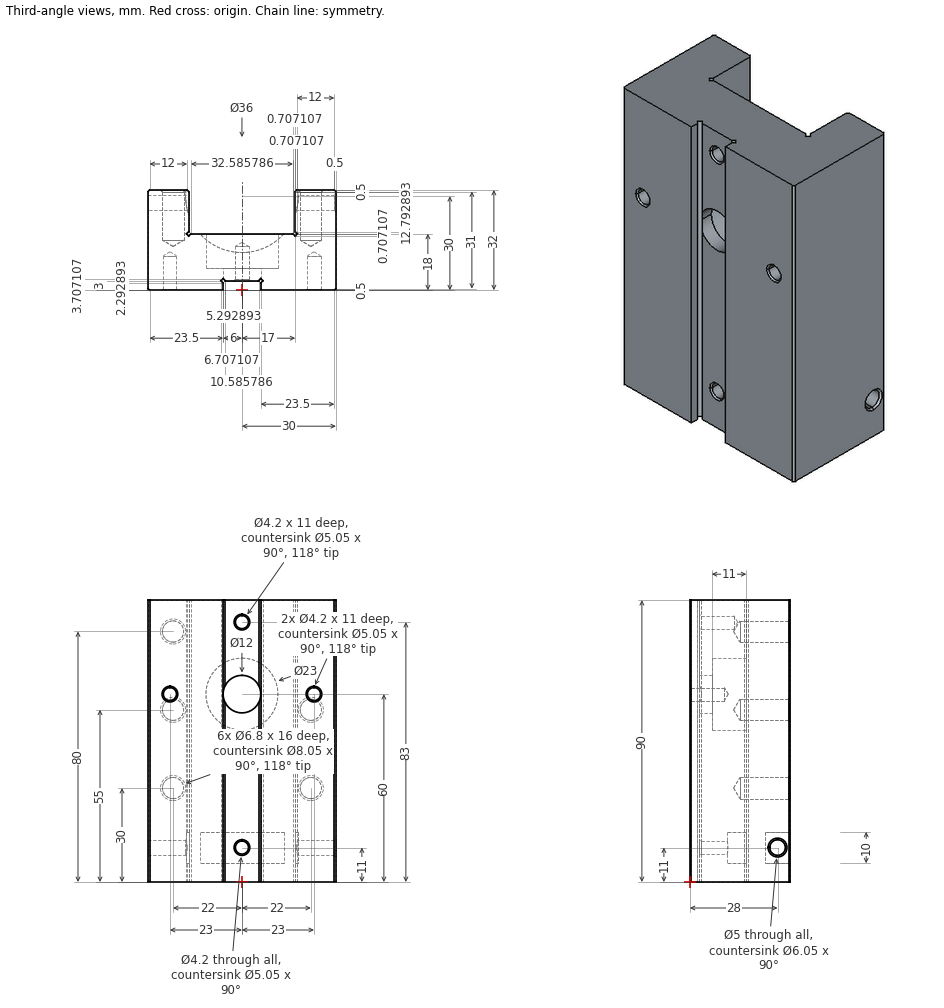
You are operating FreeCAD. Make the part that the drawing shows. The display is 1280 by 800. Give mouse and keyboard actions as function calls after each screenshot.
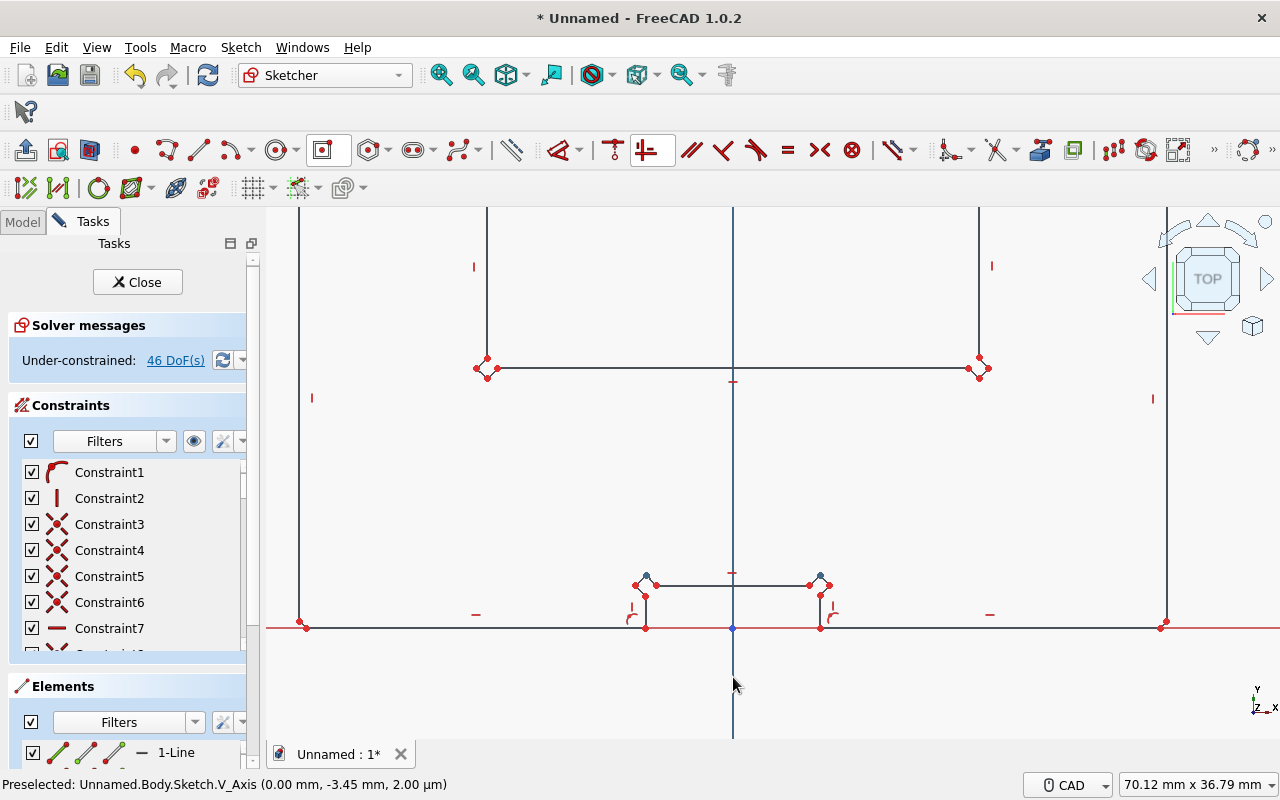
click(820, 150)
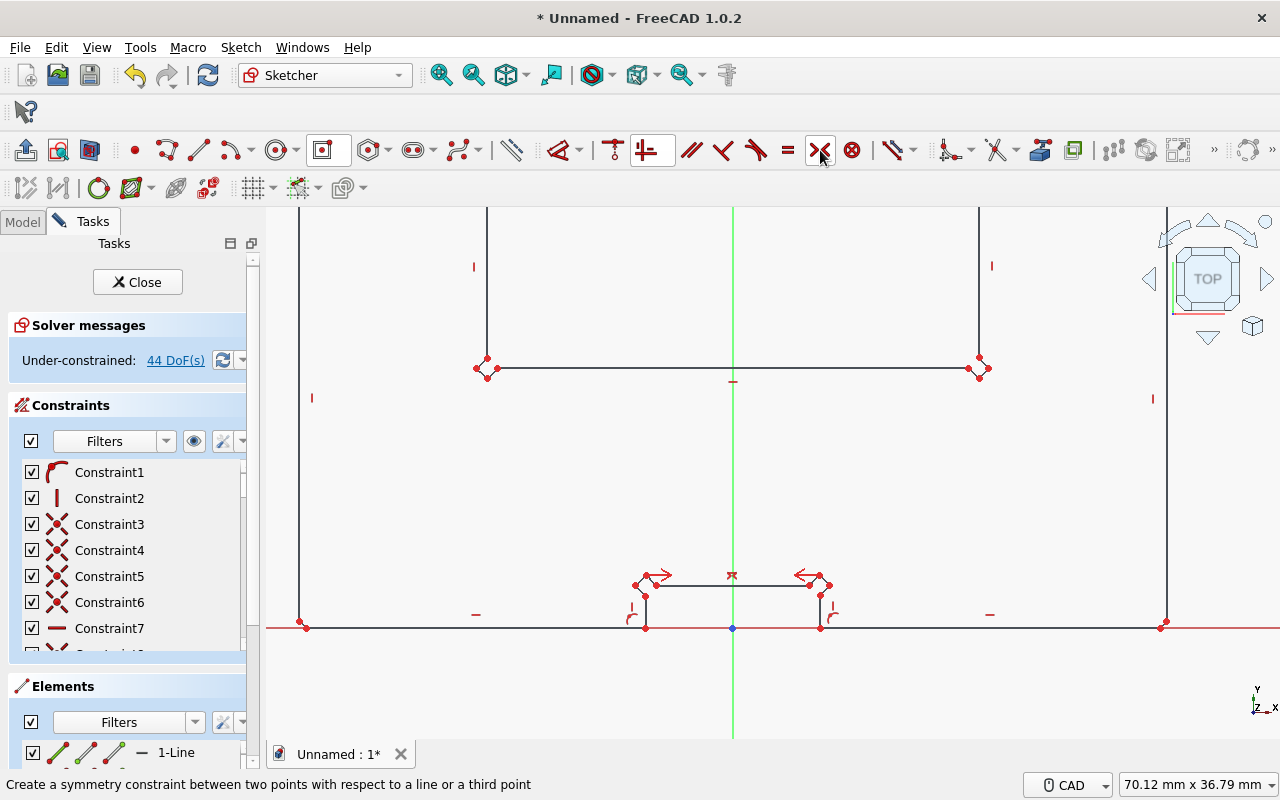
click(636, 586)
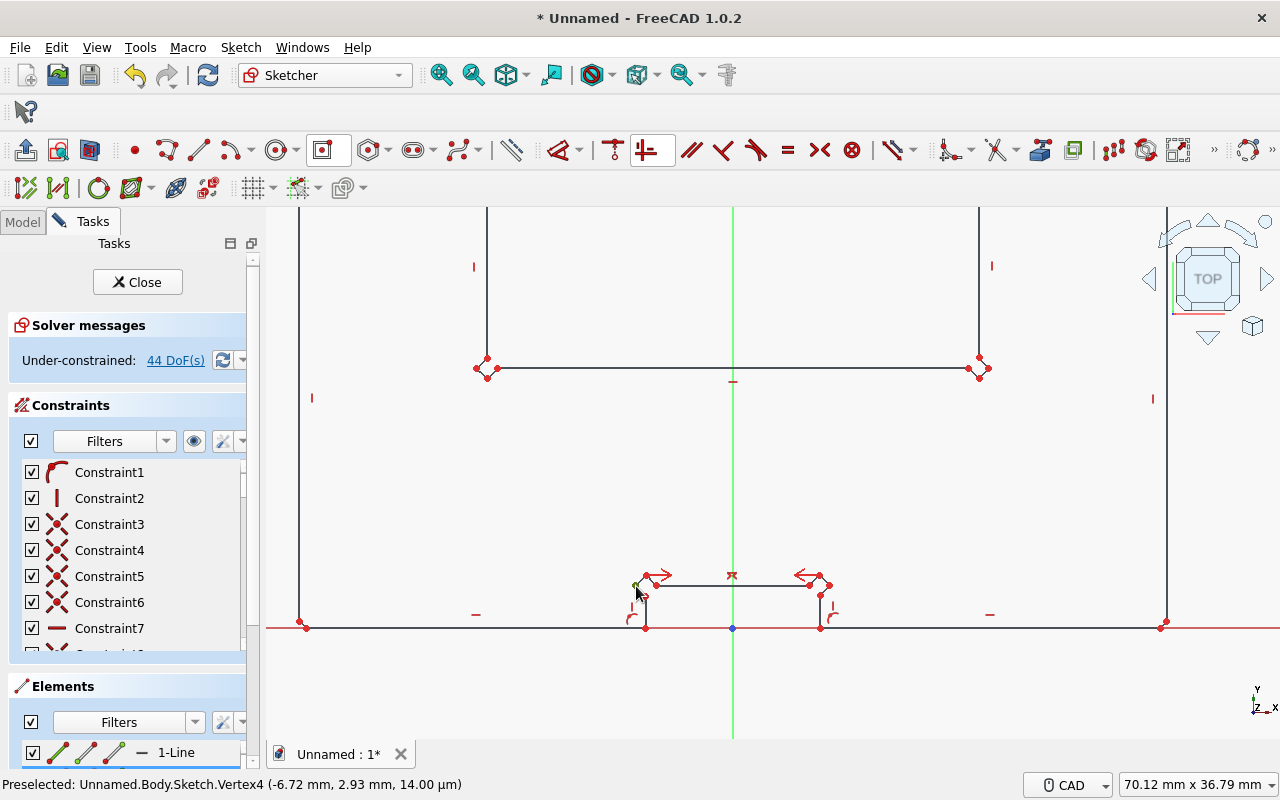
click(830, 586)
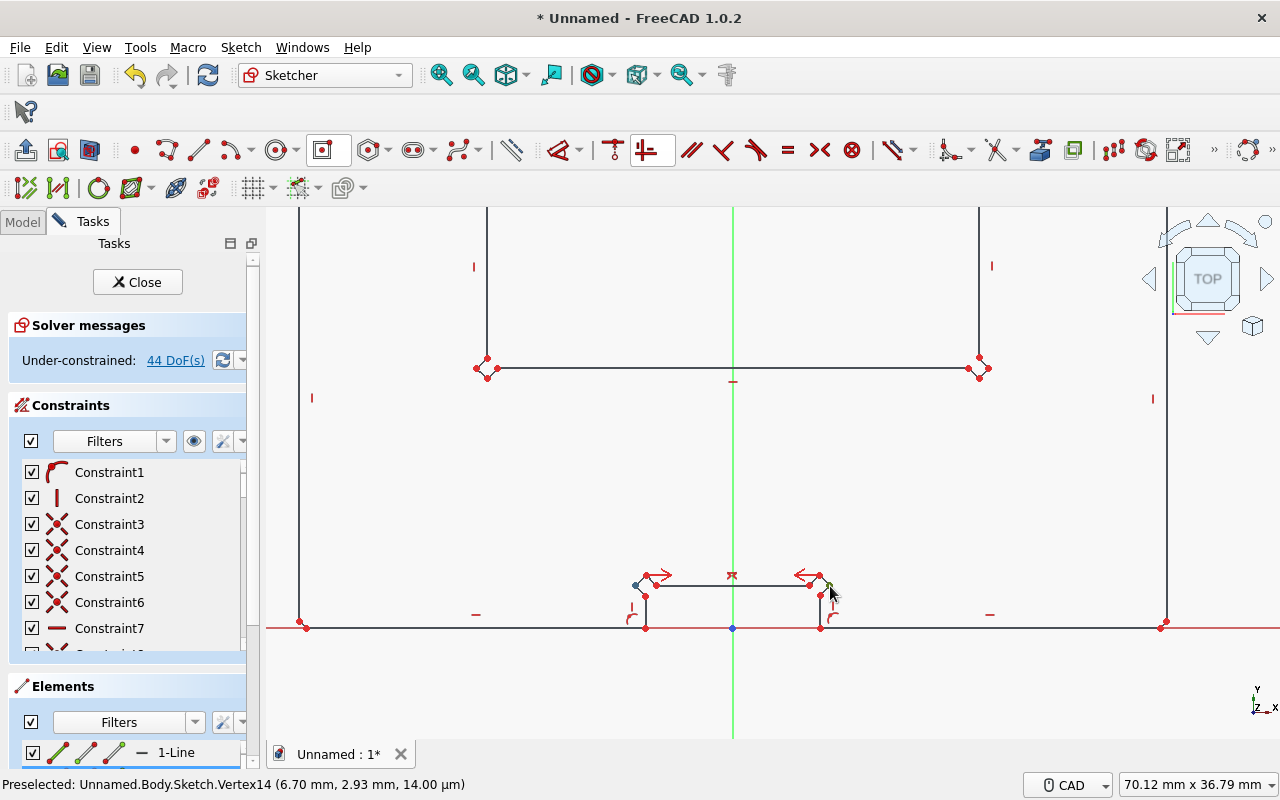
click(733, 677)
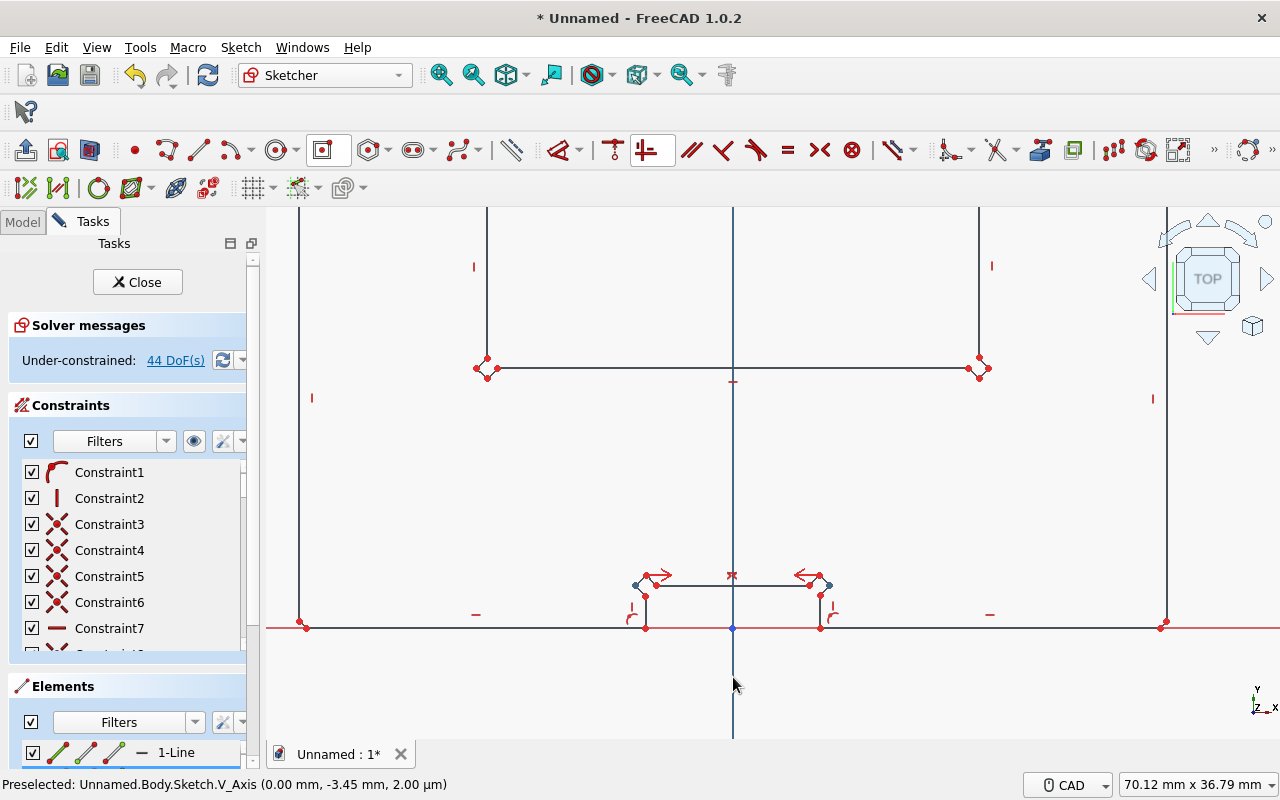
click(820, 150)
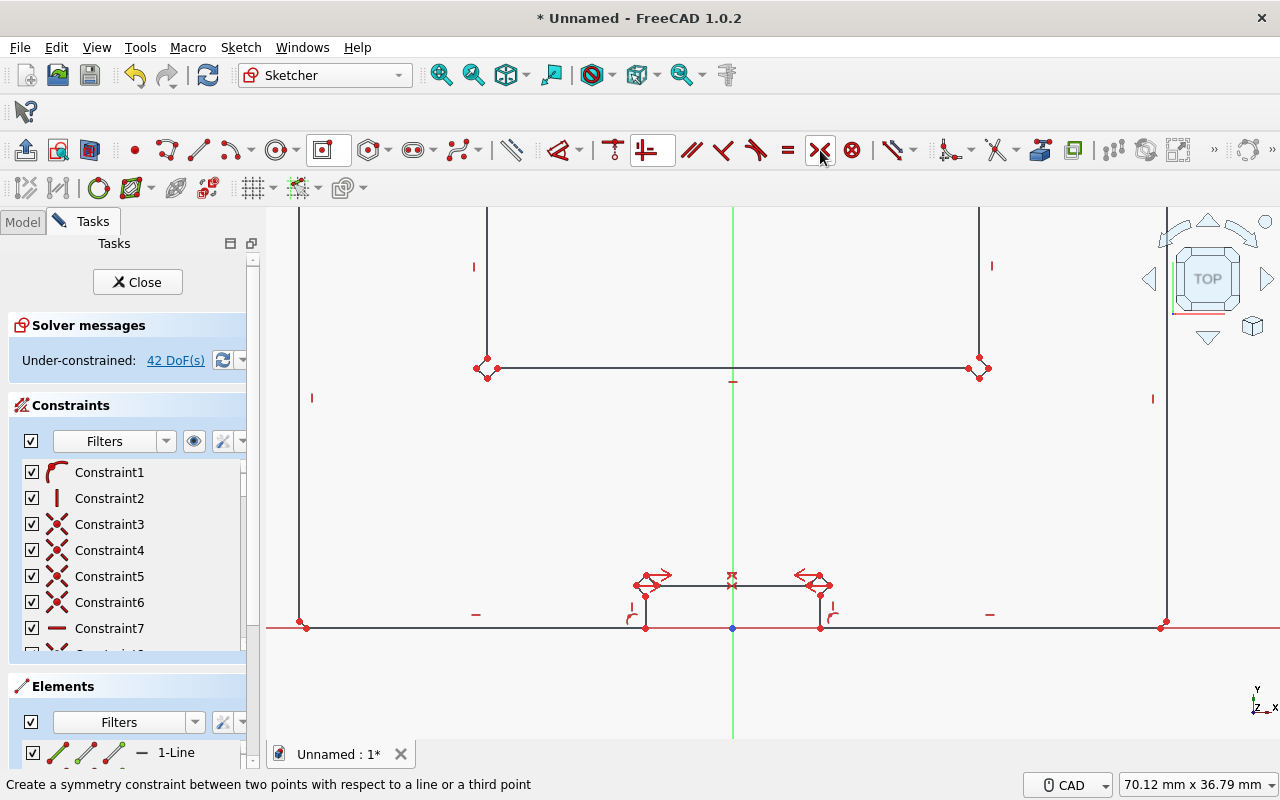
click(646, 596)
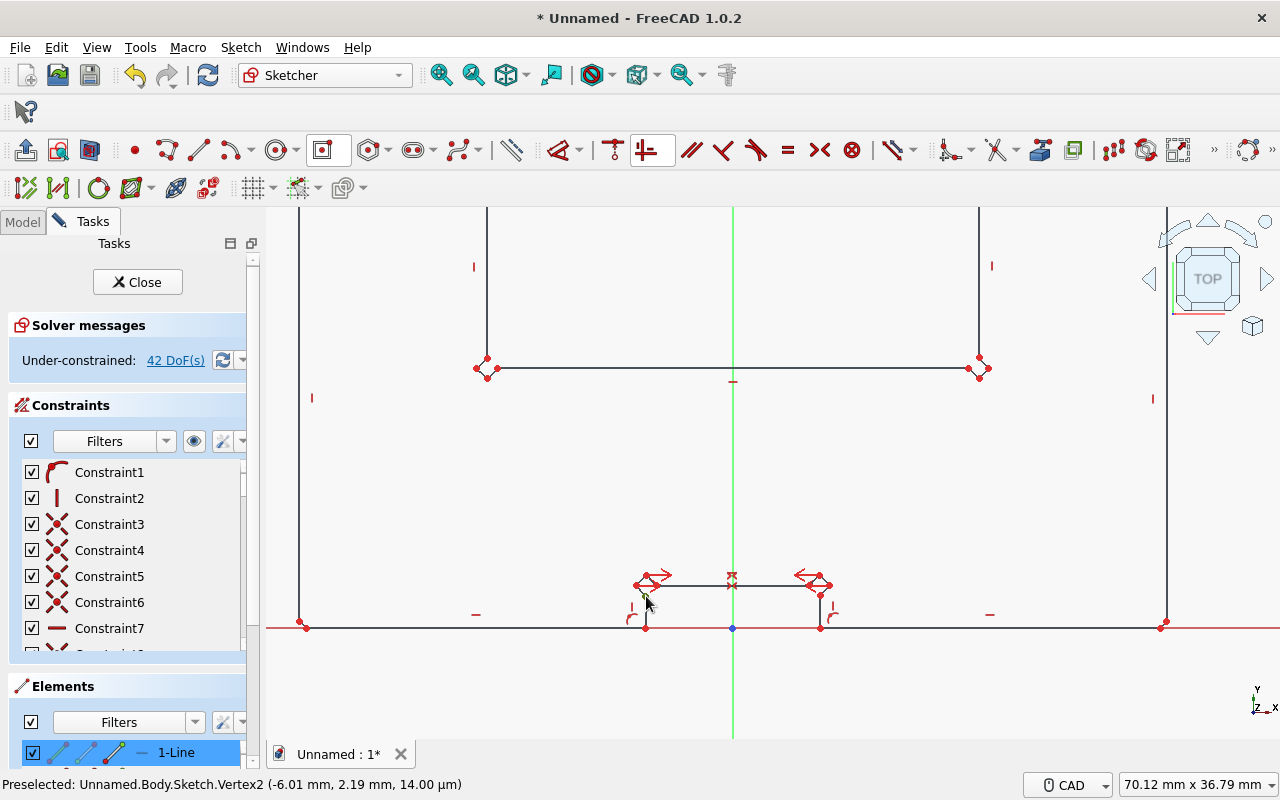
click(820, 596)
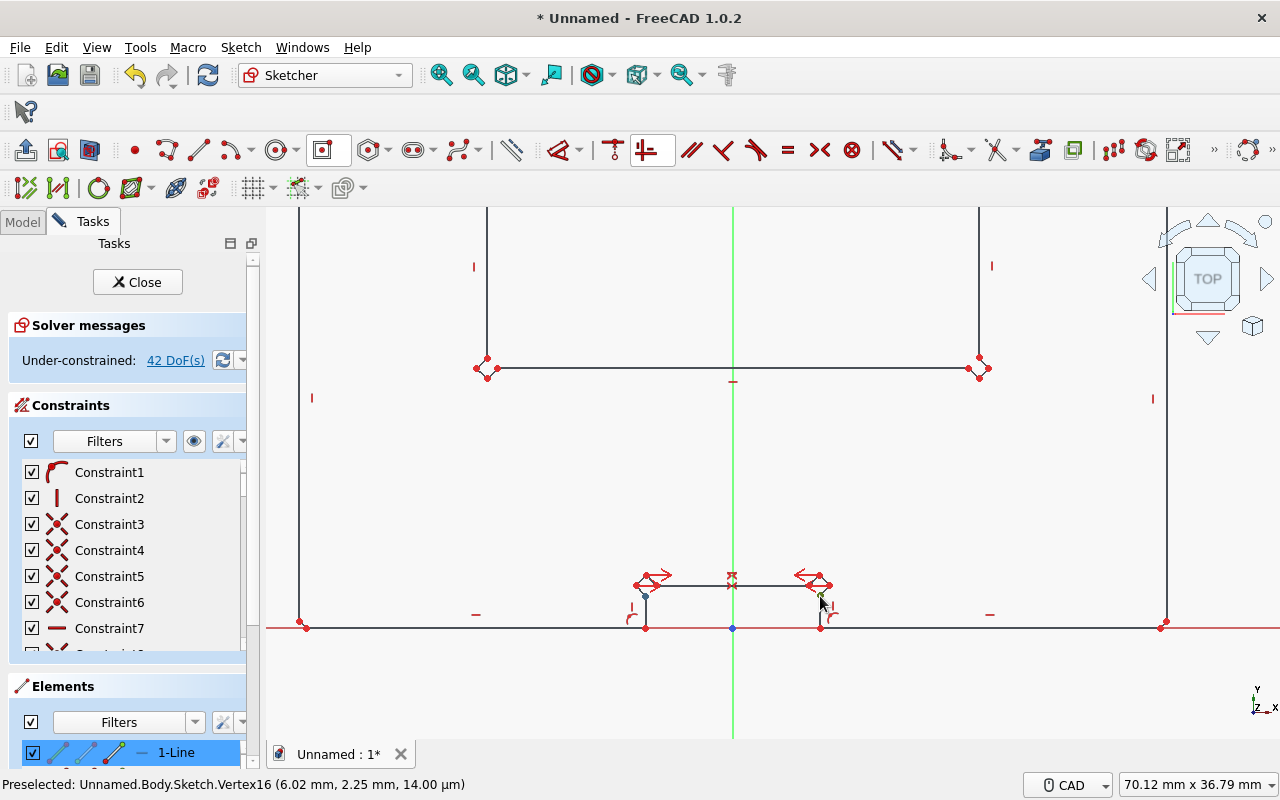
click(733, 677)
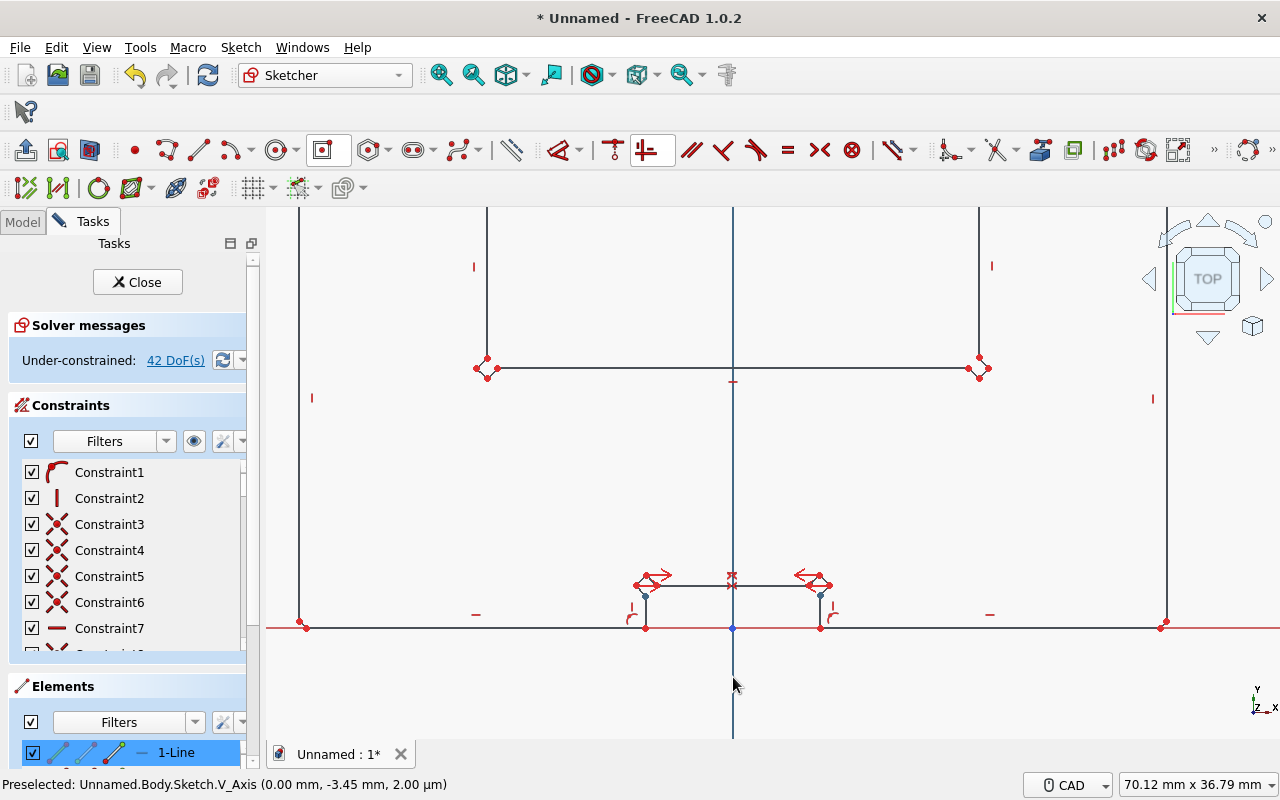
click(820, 150)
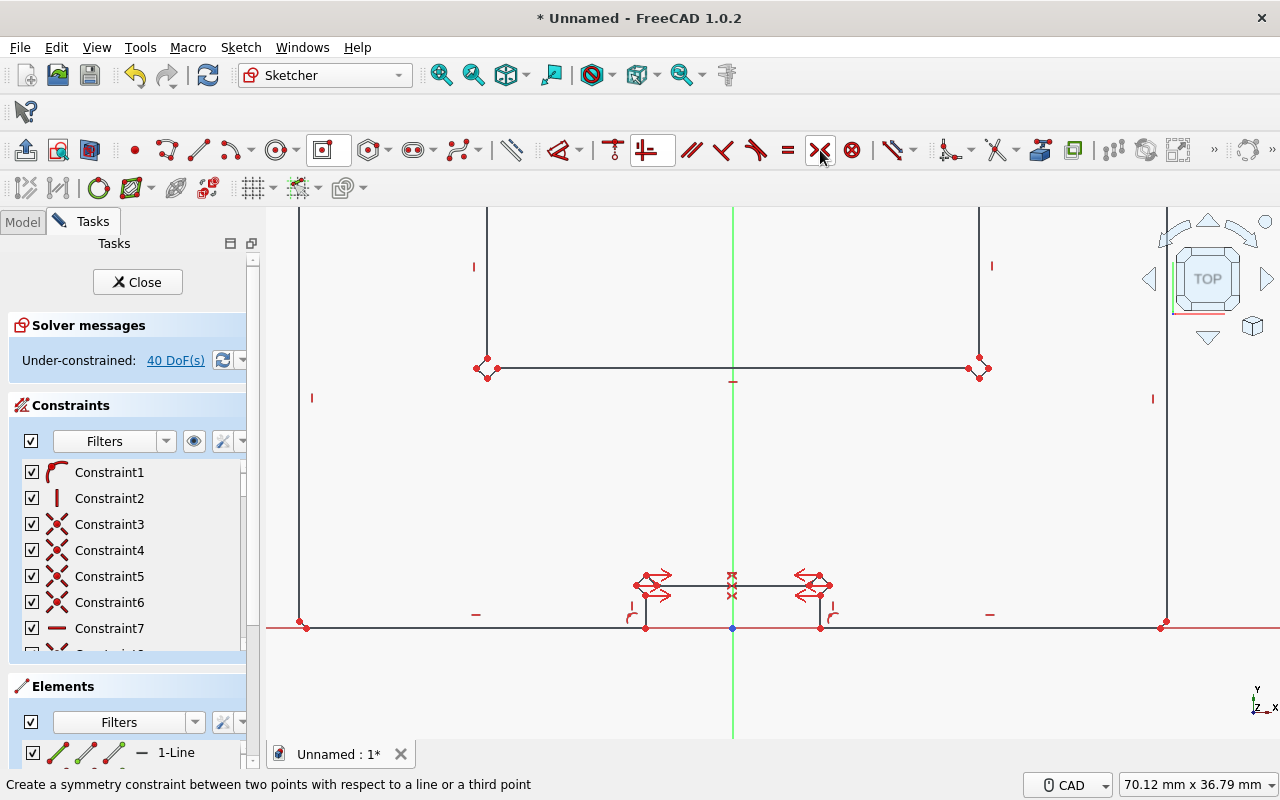
click(979, 379)